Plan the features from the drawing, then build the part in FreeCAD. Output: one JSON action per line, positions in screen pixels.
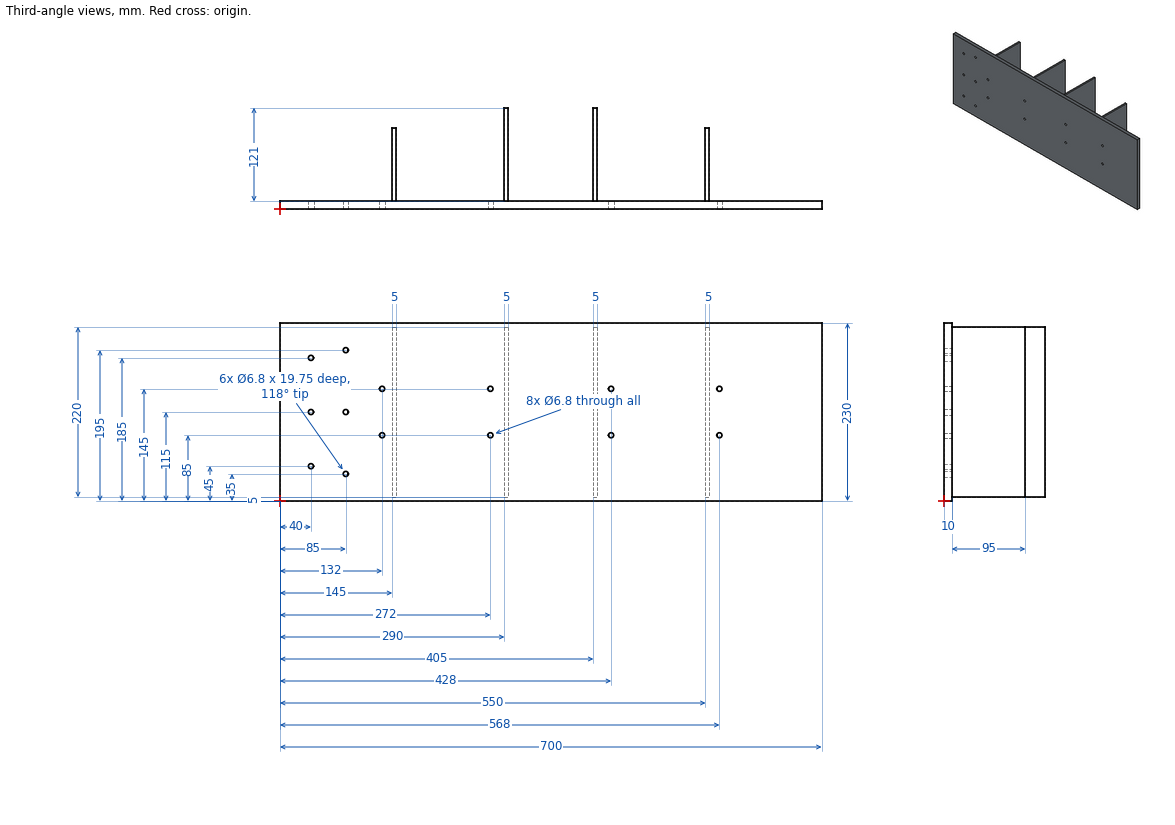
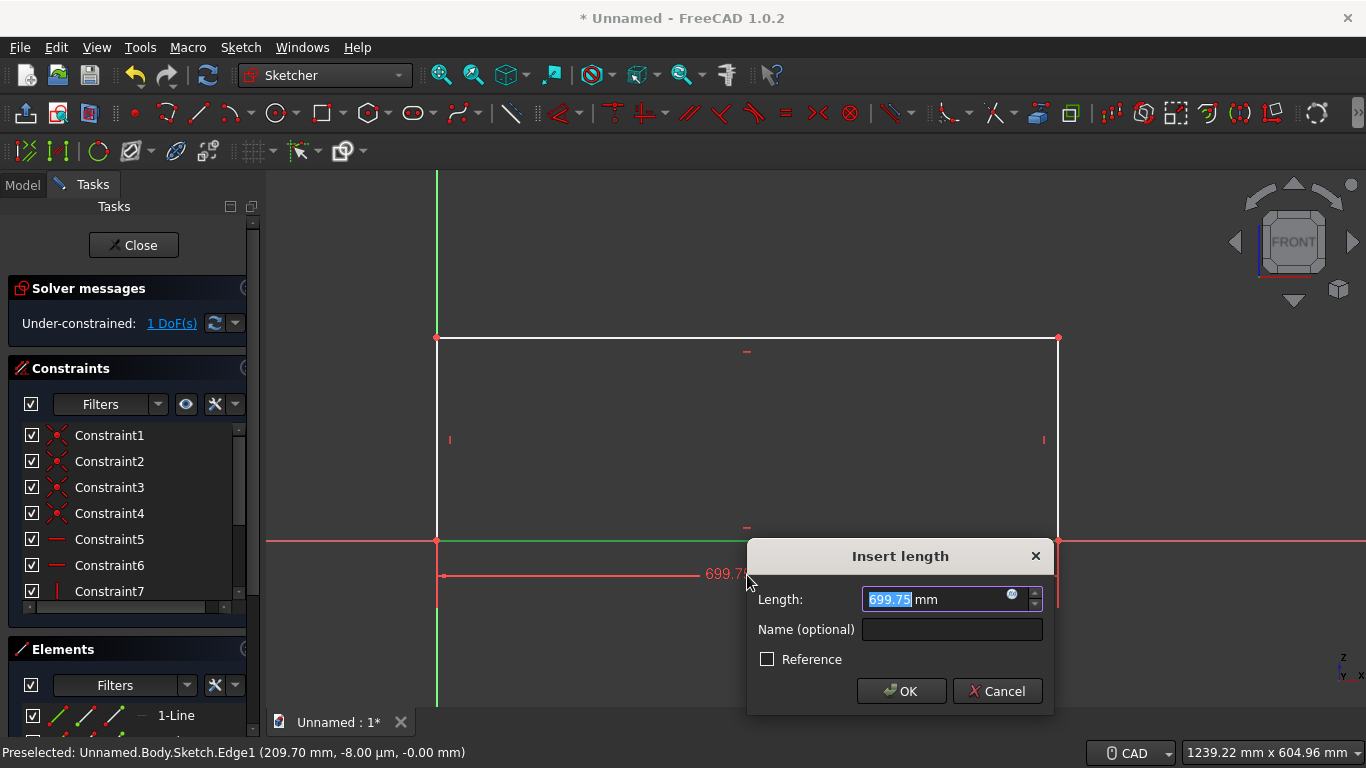
{"action": "type", "text": "700"}
{"action": "key", "text": "Return"}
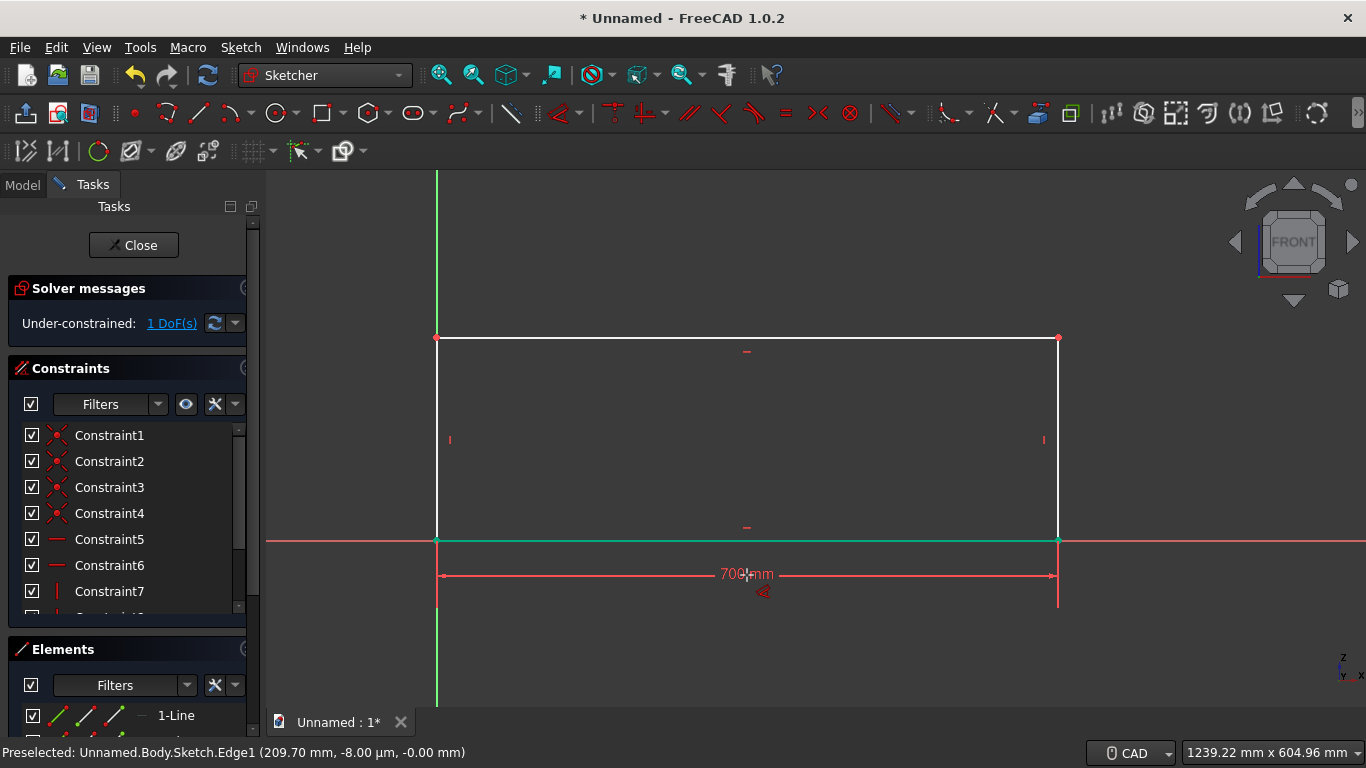
{"action": "left_click", "coordinate": [1058, 480]}
{"action": "left_click", "coordinate": [1092, 439]}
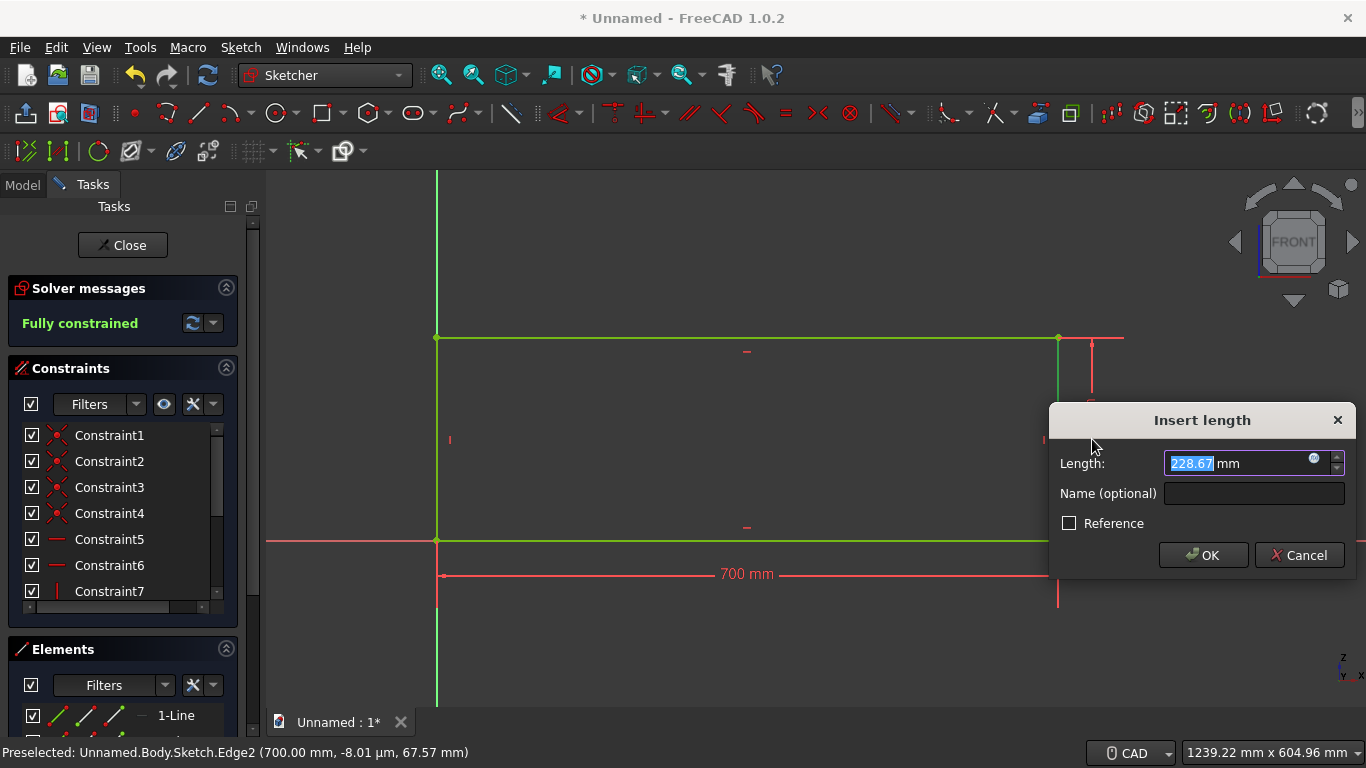
{"action": "type", "text": "230"}
{"action": "key", "text": "Return"}
{"action": "key", "text": "Escape"}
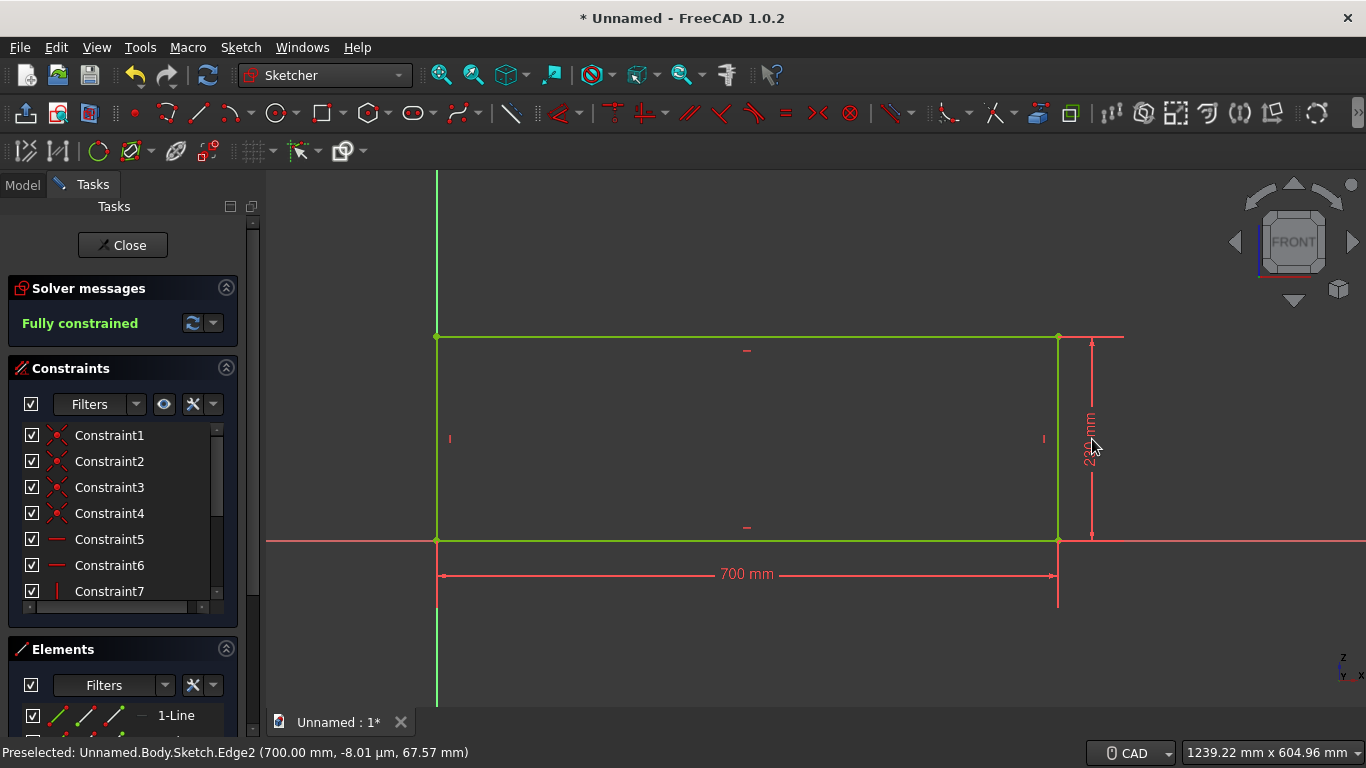
{"action": "left_click", "coordinate": [123, 245]}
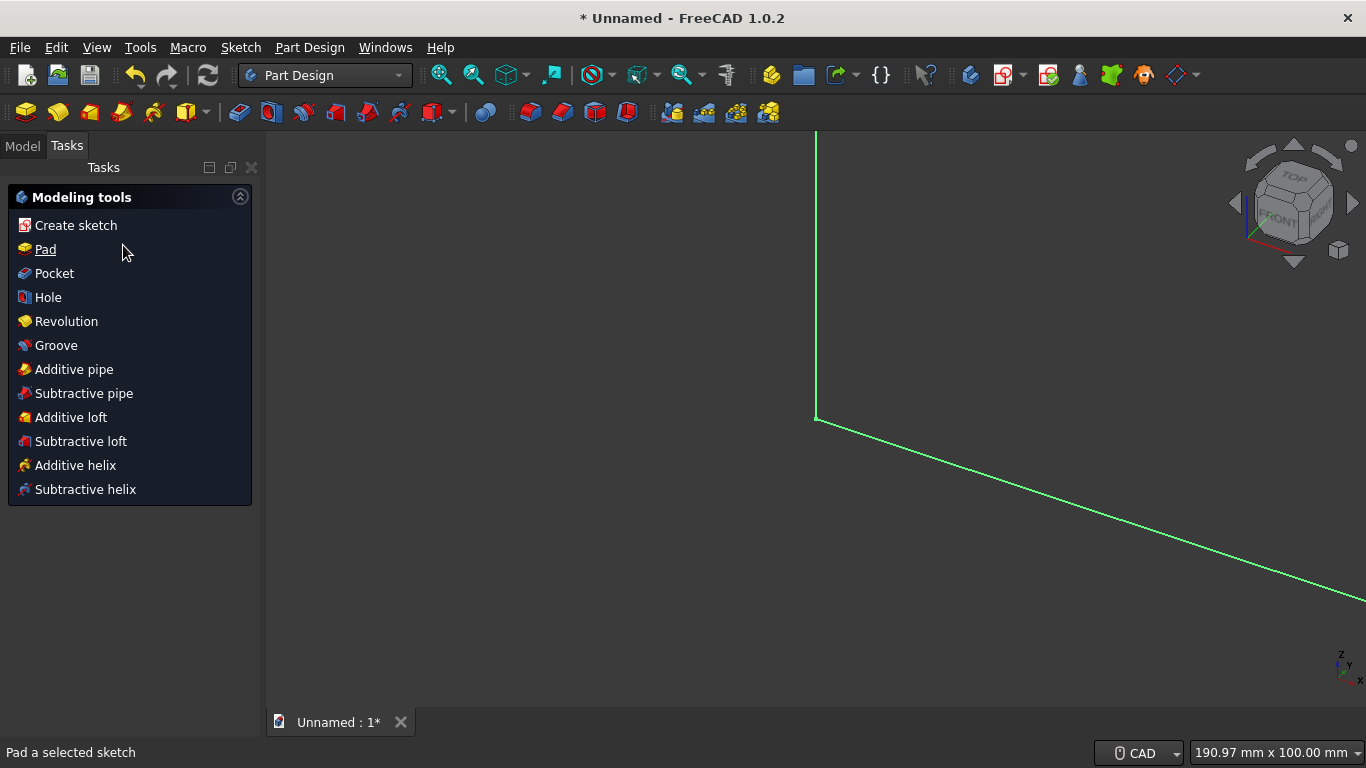
{"action": "left_click", "coordinate": [26, 112]}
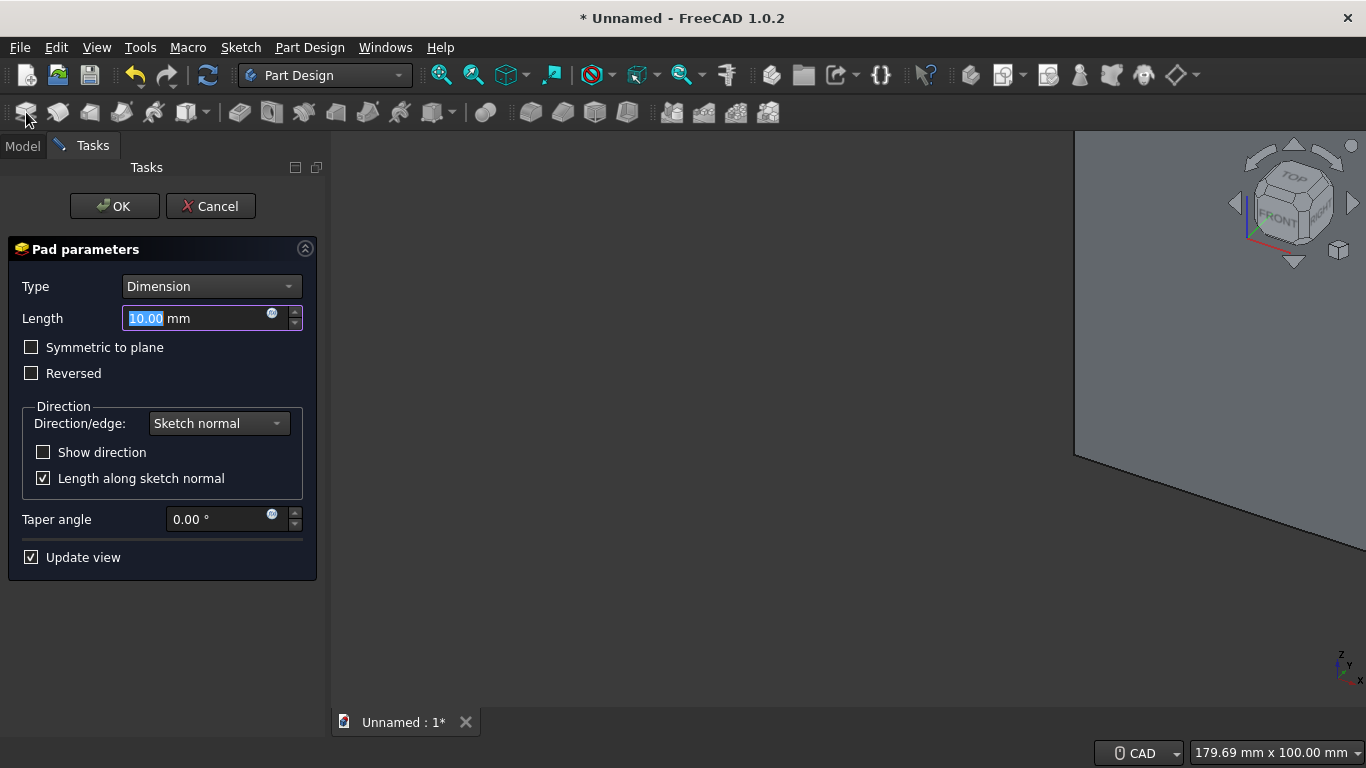
{"action": "type", "text": "10"}
{"action": "key", "text": "Tab"}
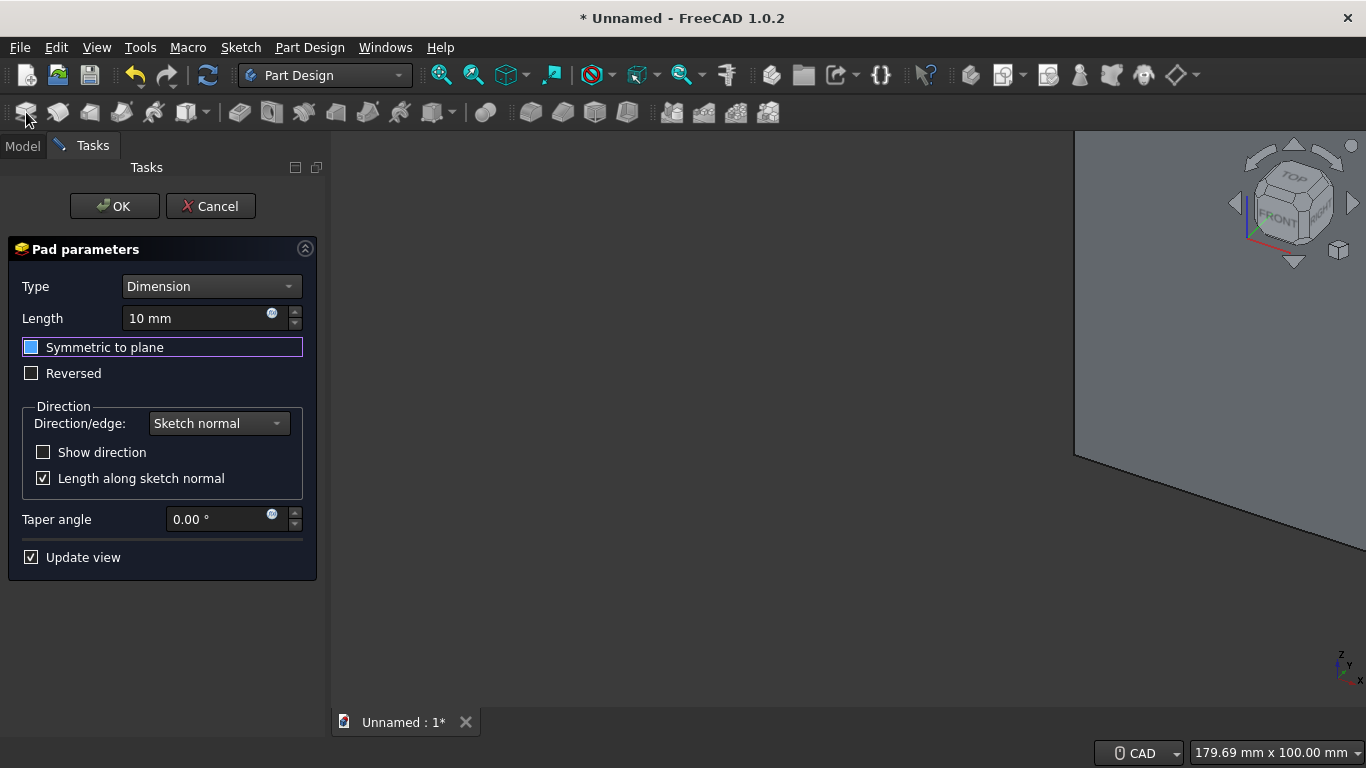
{"action": "left_click", "coordinate": [30, 373]}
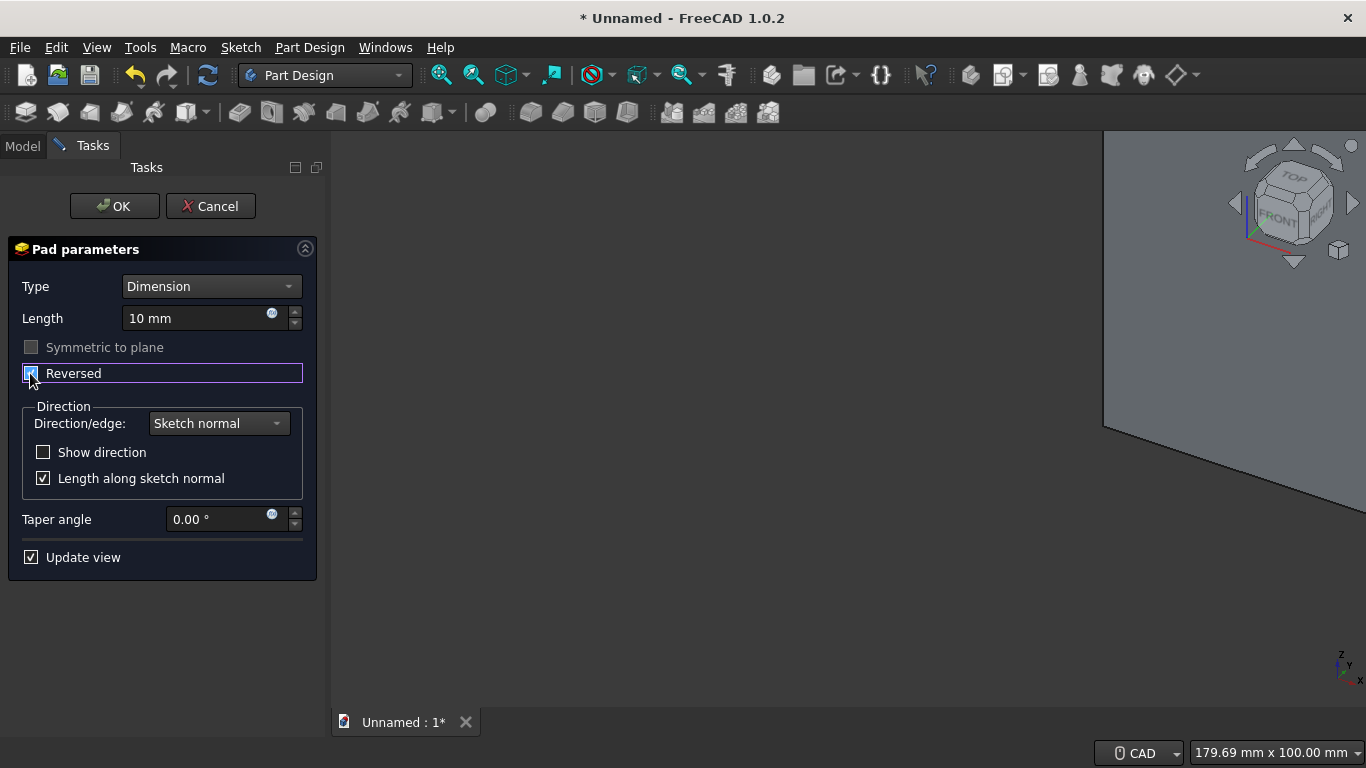
{"action": "left_click", "coordinate": [115, 206]}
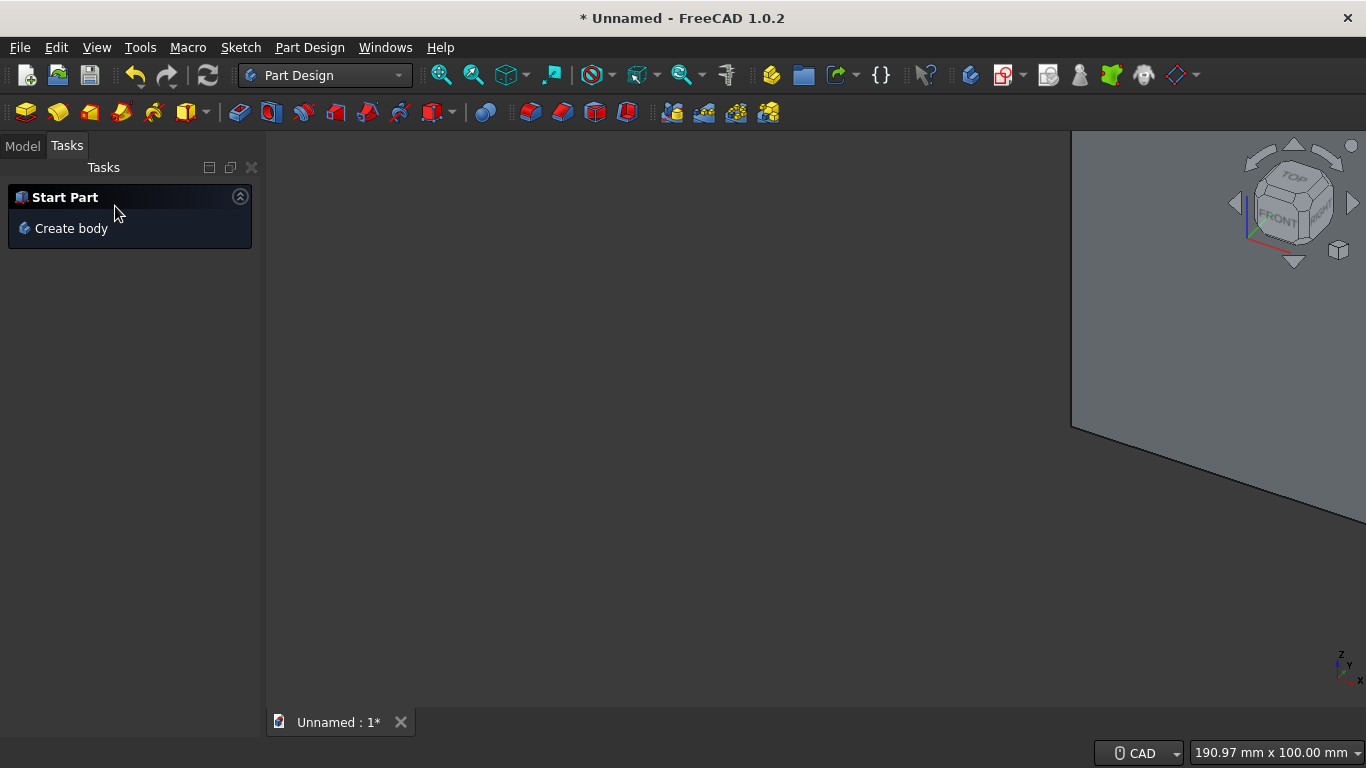
{"action": "key", "text": "v f"}